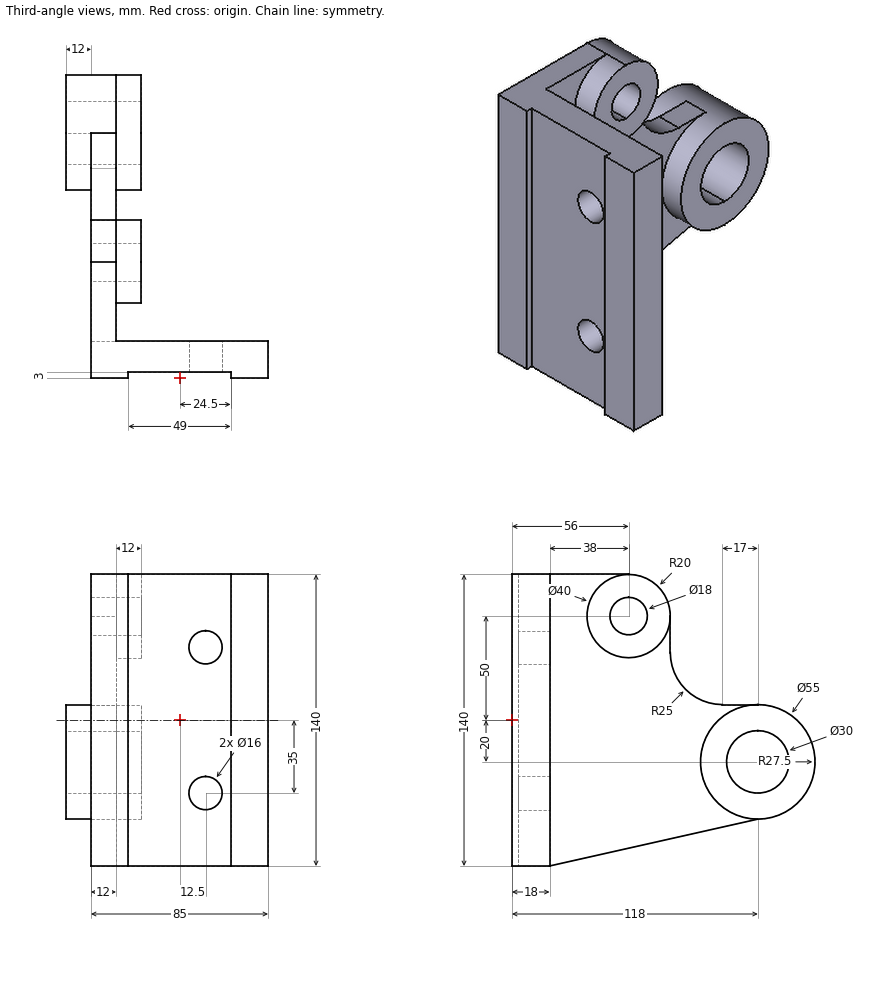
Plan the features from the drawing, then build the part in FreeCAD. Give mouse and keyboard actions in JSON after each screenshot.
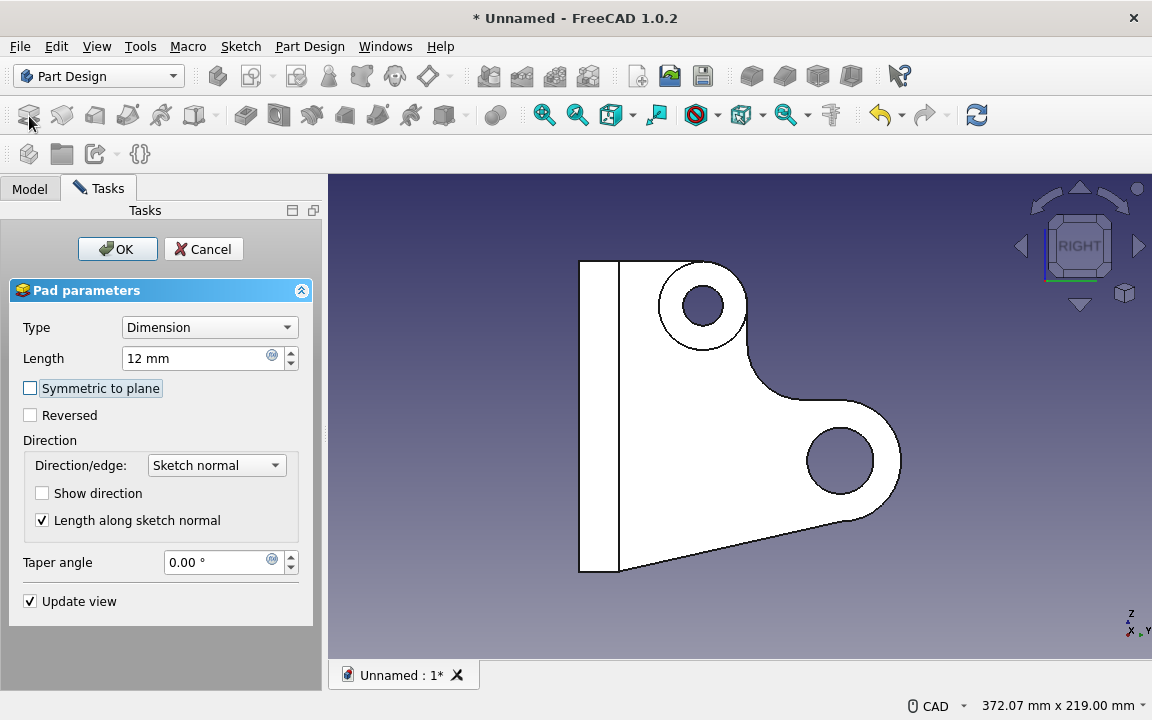
{"action": "left_click", "coordinate": [118, 249]}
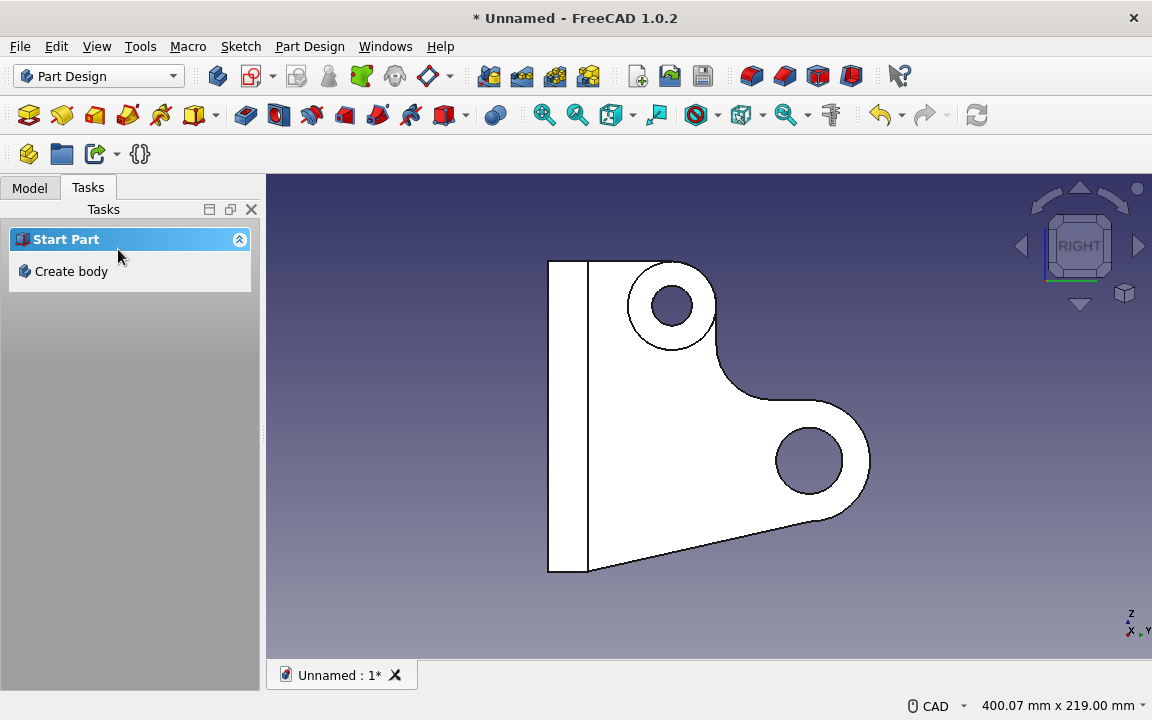
{"action": "left_click", "coordinate": [30, 188]}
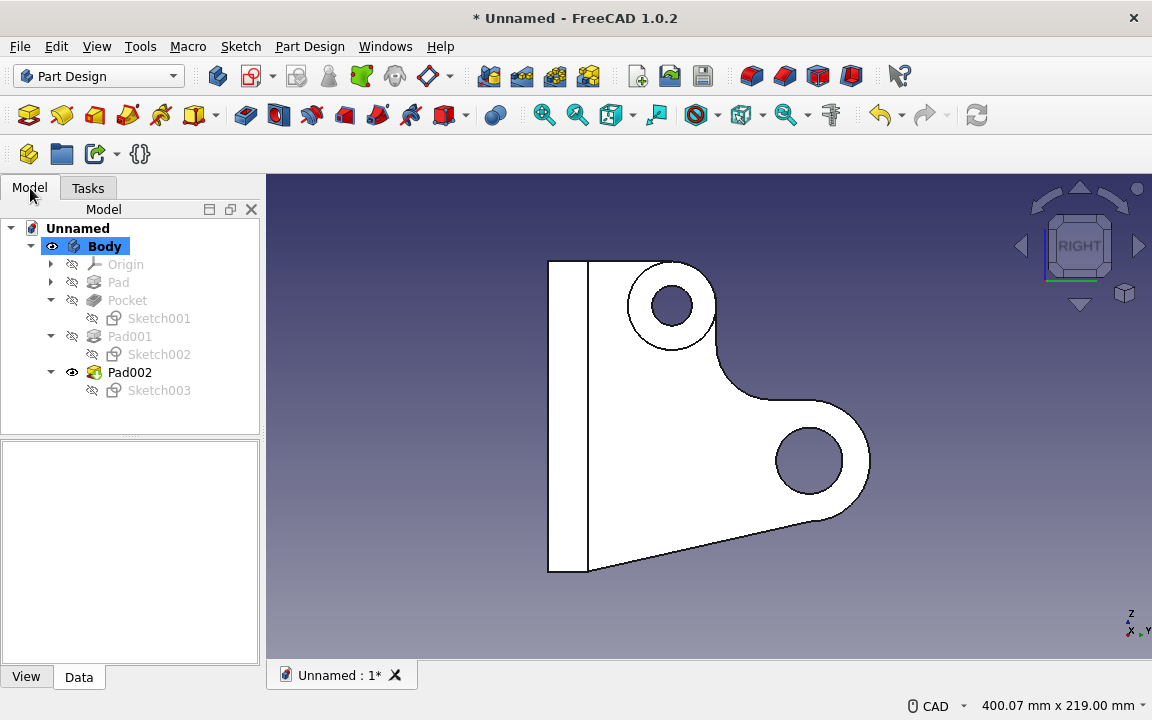
{"action": "left_click", "coordinate": [51, 264]}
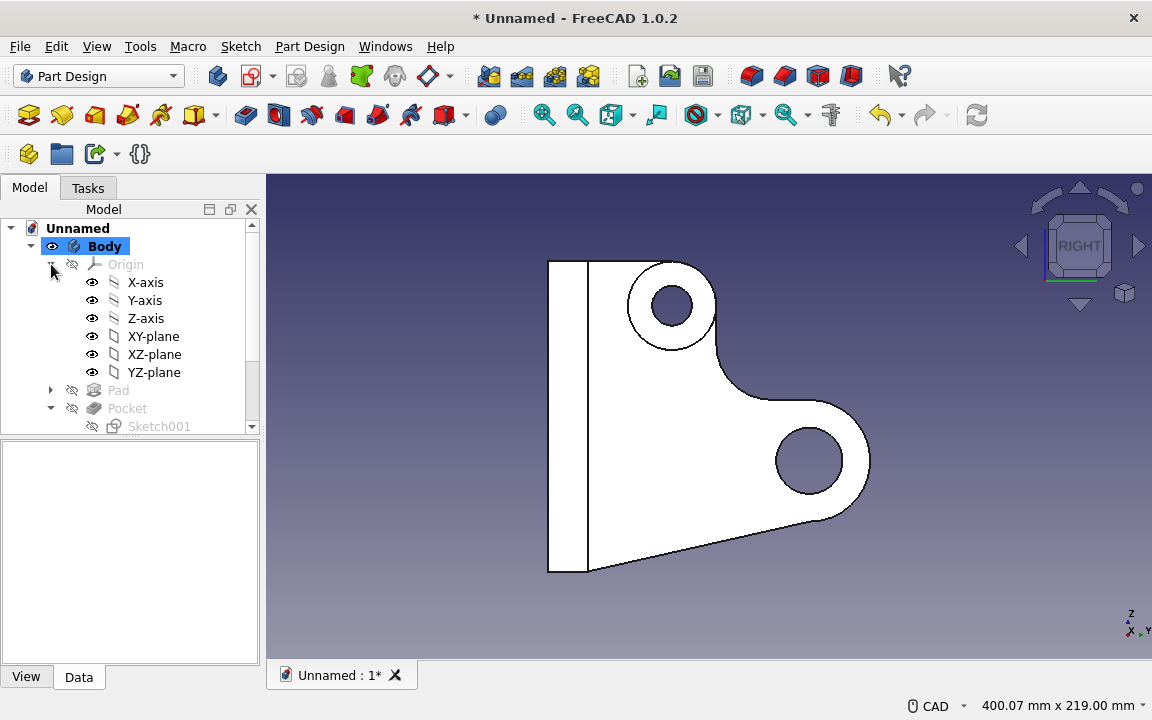
{"action": "left_click", "coordinate": [137, 372]}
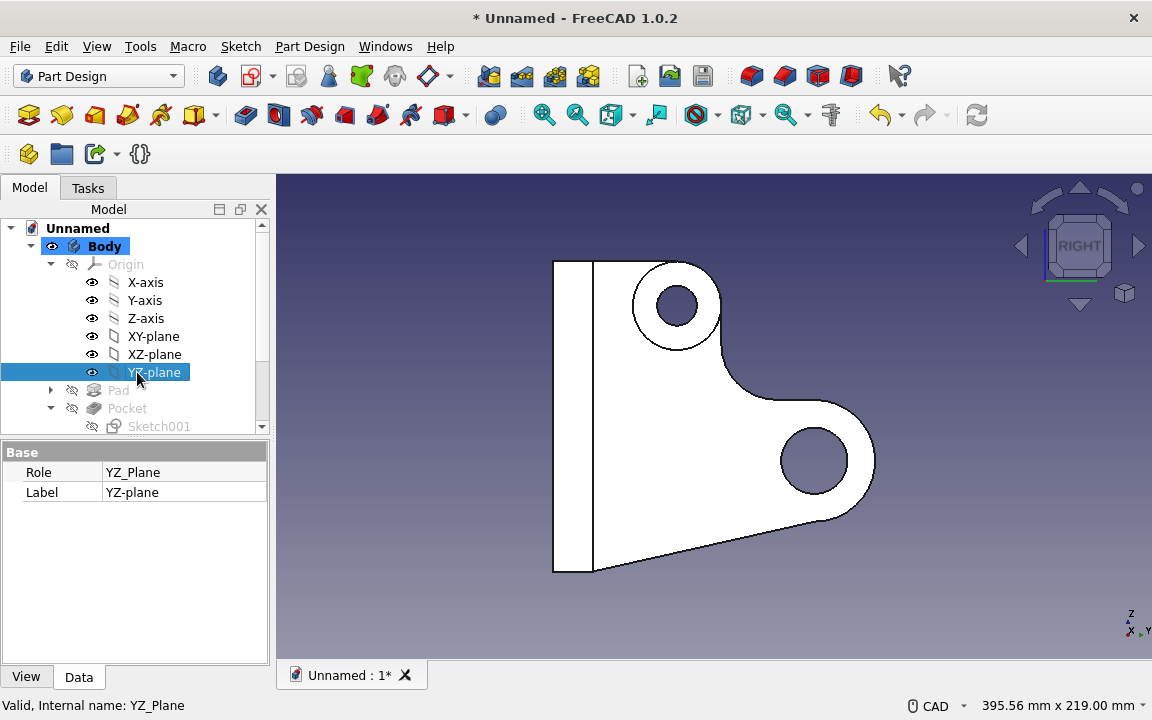
{"action": "left_click", "coordinate": [428, 76]}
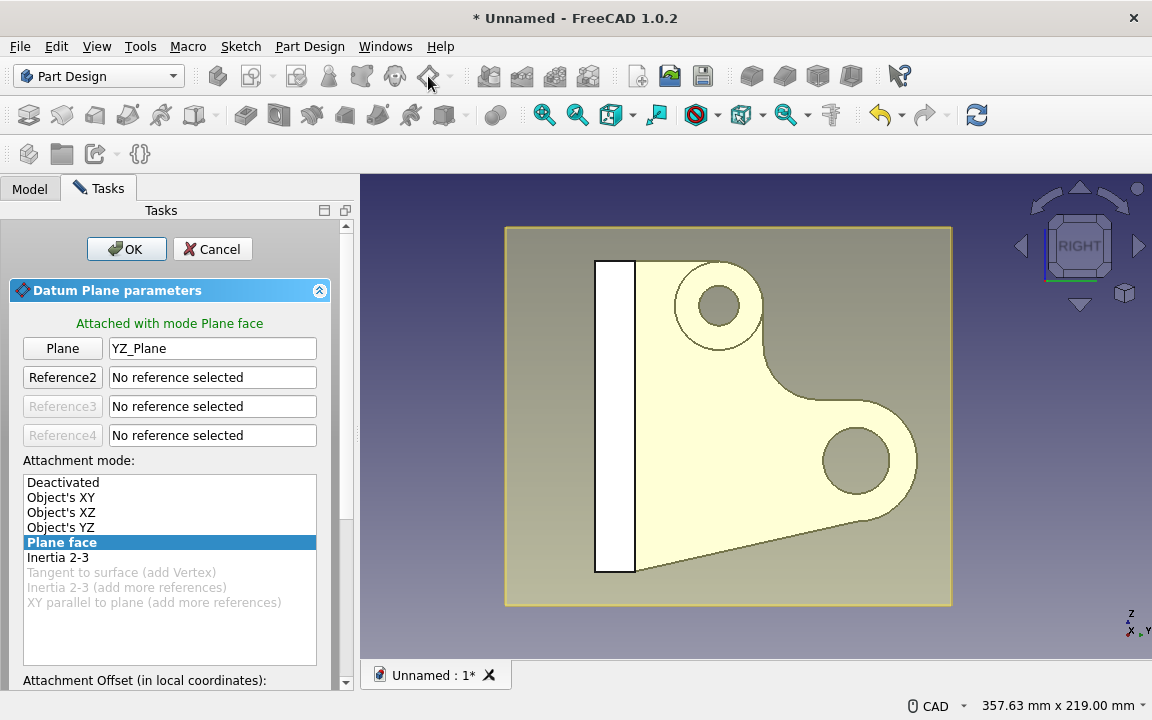
{"action": "scroll", "coordinate": [346, 455], "scroll_direction": "down", "scroll_amount": 3}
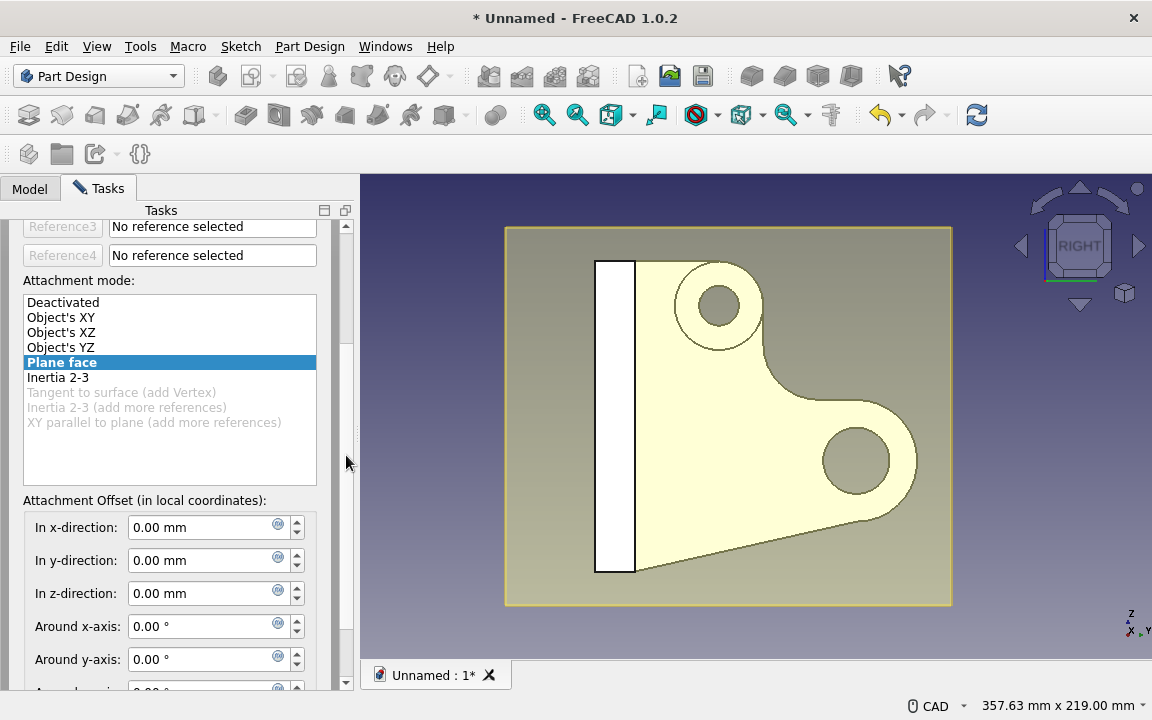
{"action": "triple_click", "coordinate": [210, 594]}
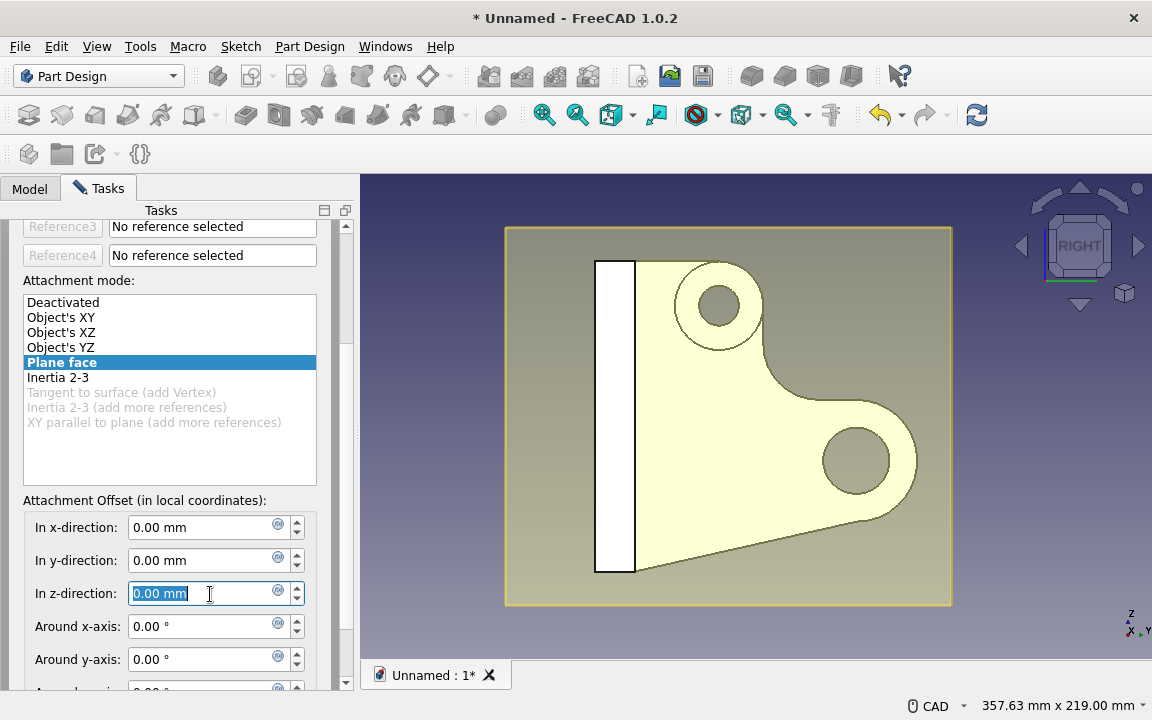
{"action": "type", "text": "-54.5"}
{"action": "key", "text": "Tab"}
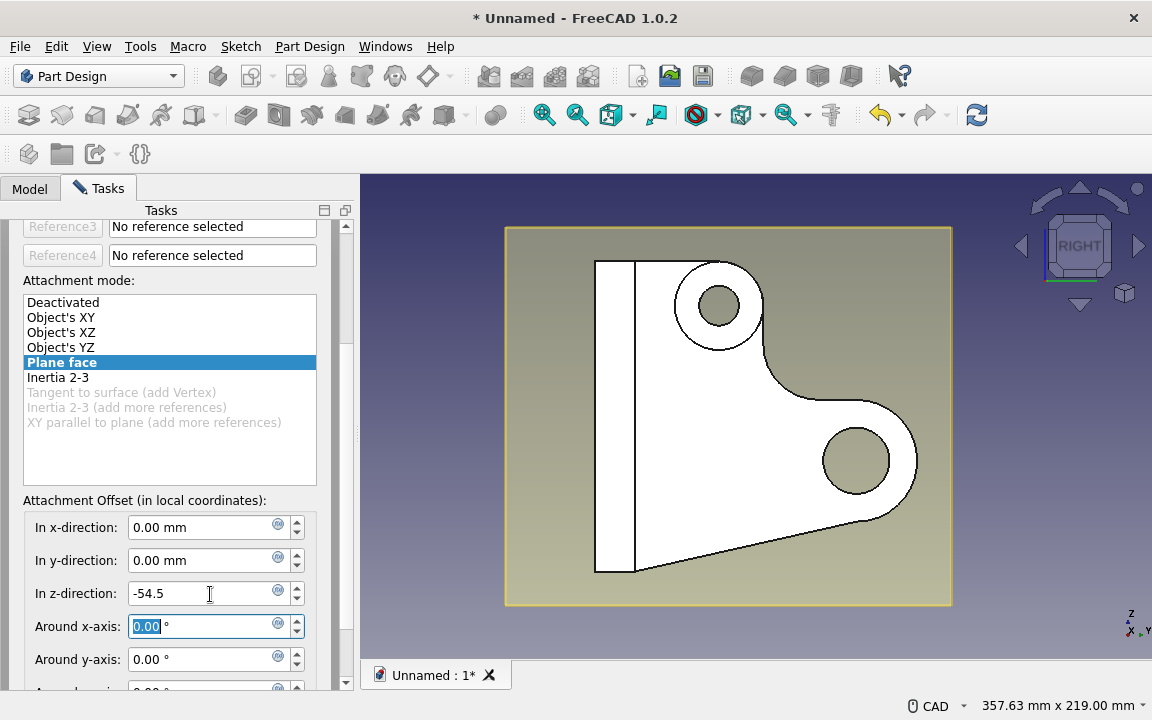
{"action": "scroll", "coordinate": [346, 455], "scroll_direction": "up", "scroll_amount": 4}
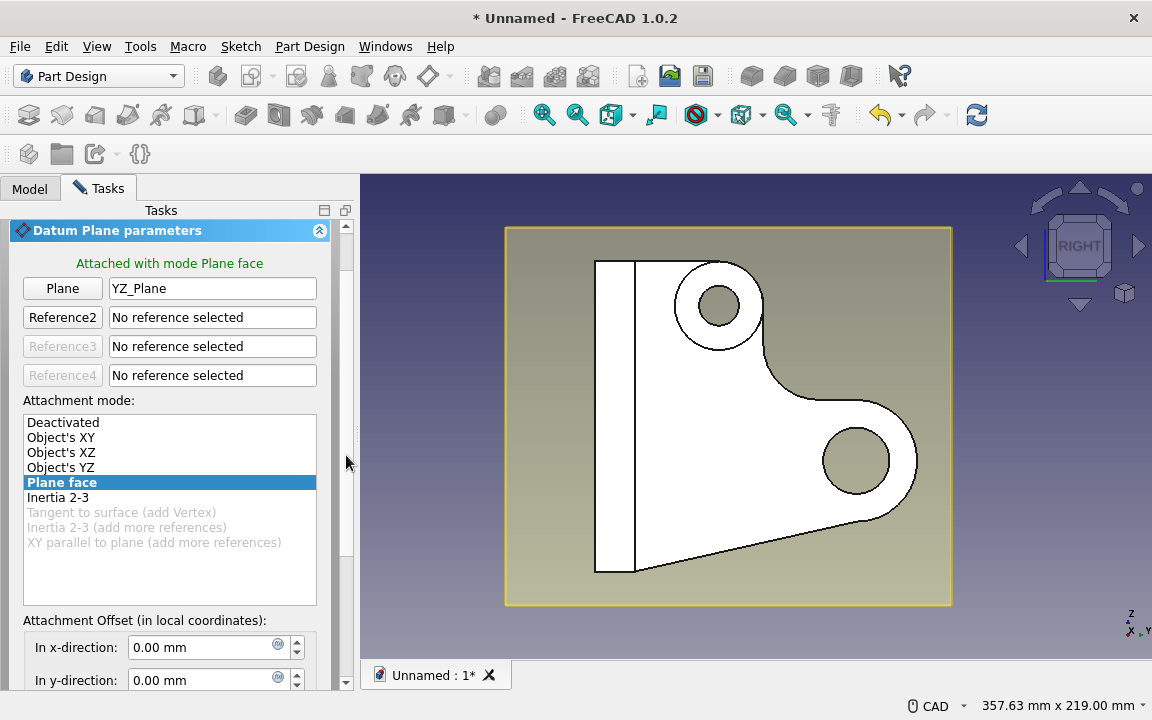
{"action": "left_click", "coordinate": [127, 249]}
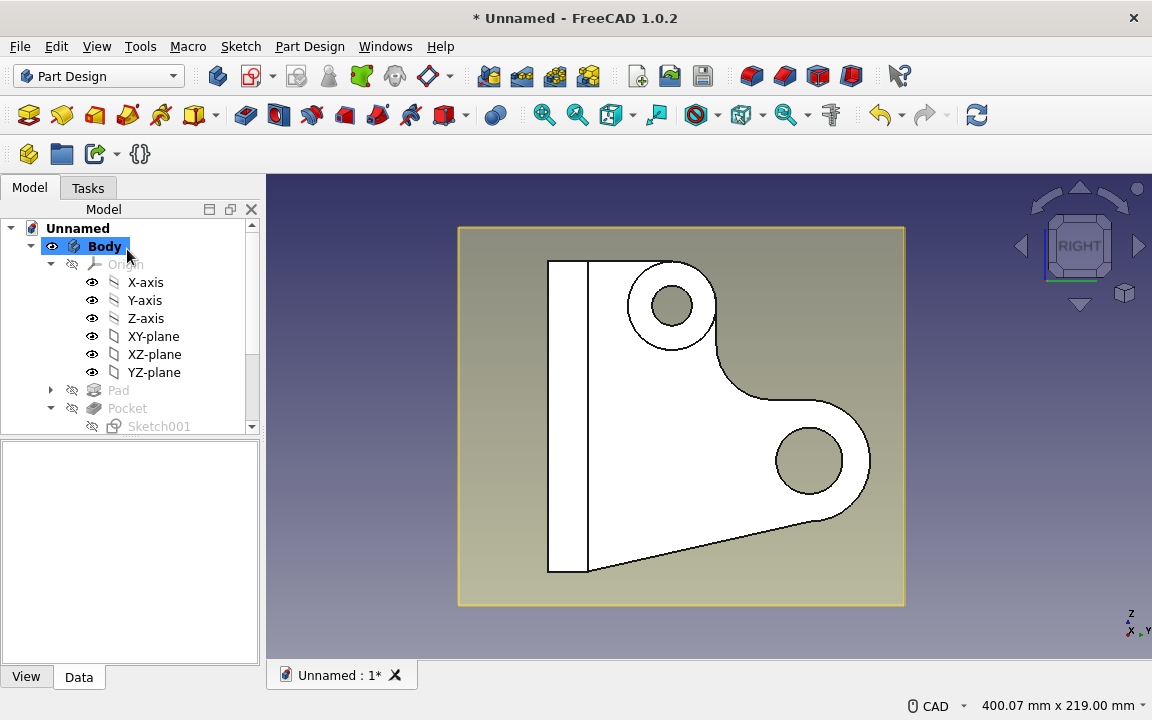
{"action": "scroll", "coordinate": [101, 332], "scroll_direction": "down", "scroll_amount": 3}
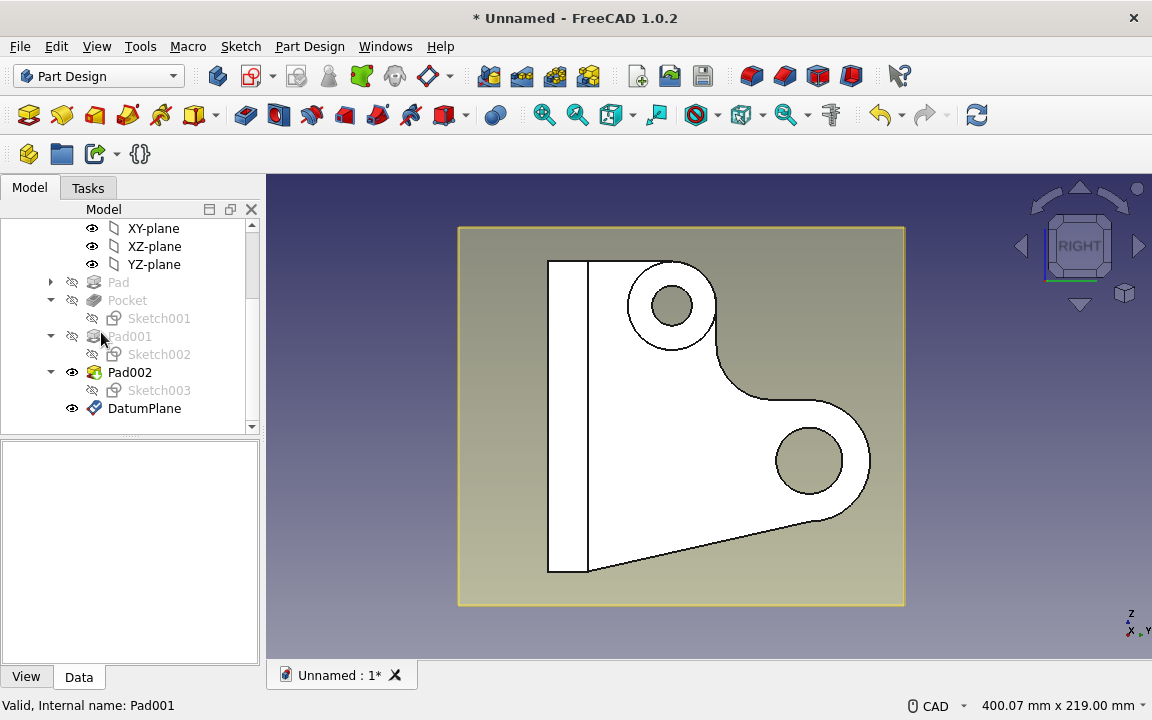
{"action": "left_click", "coordinate": [117, 408]}